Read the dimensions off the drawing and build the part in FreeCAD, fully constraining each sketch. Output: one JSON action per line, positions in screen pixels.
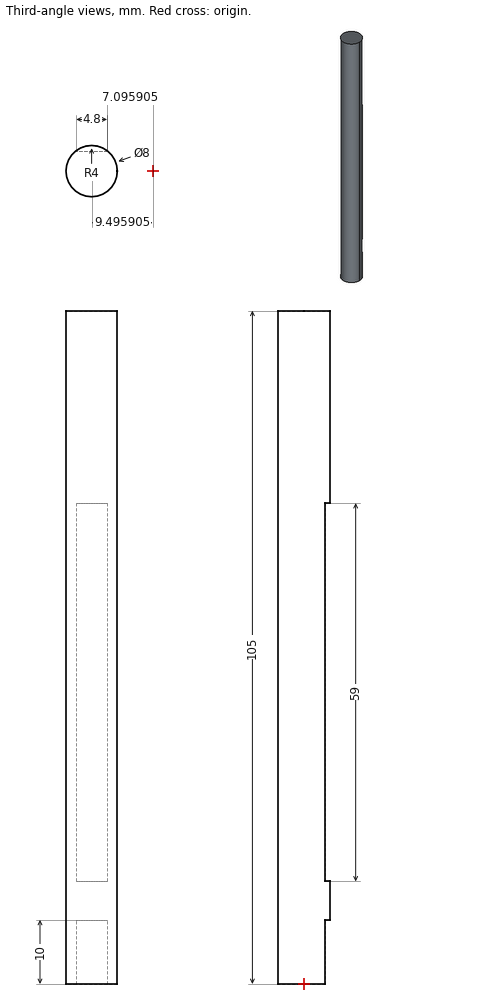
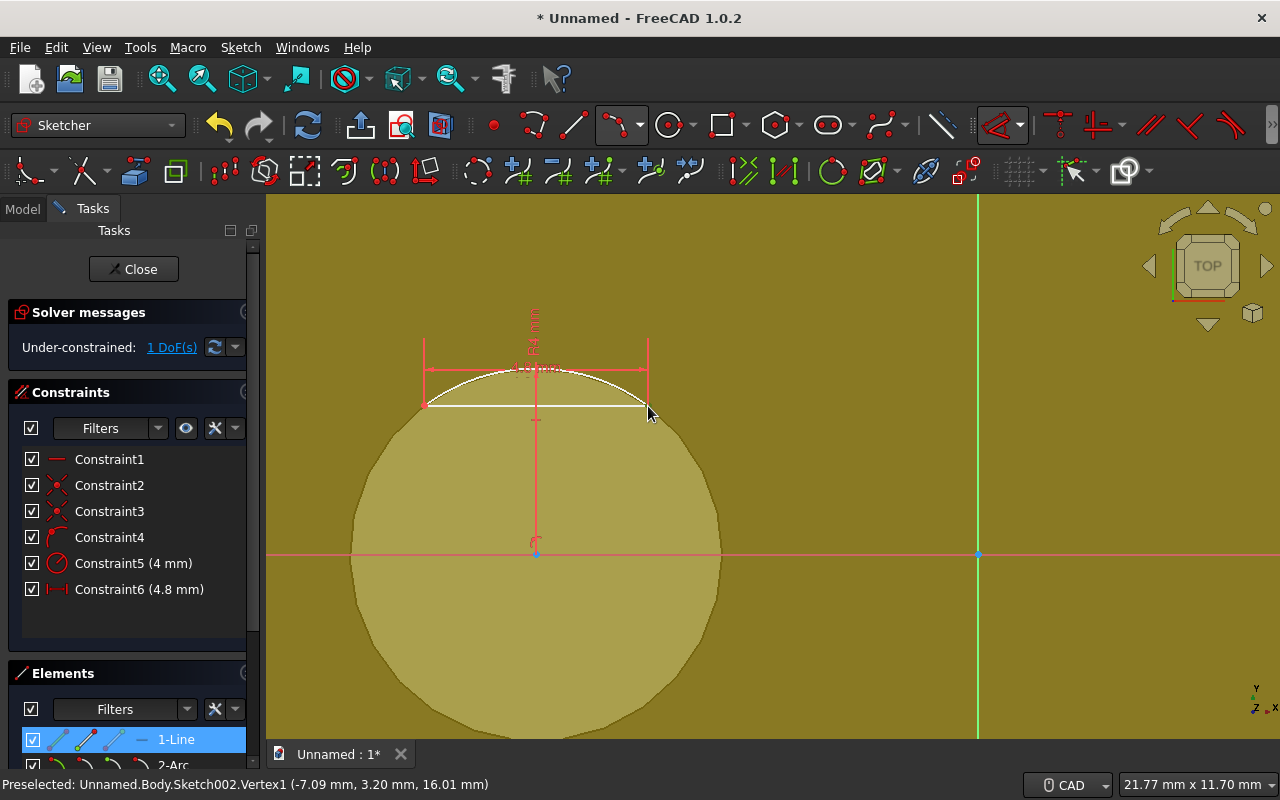
{"action": "key", "text": "l"}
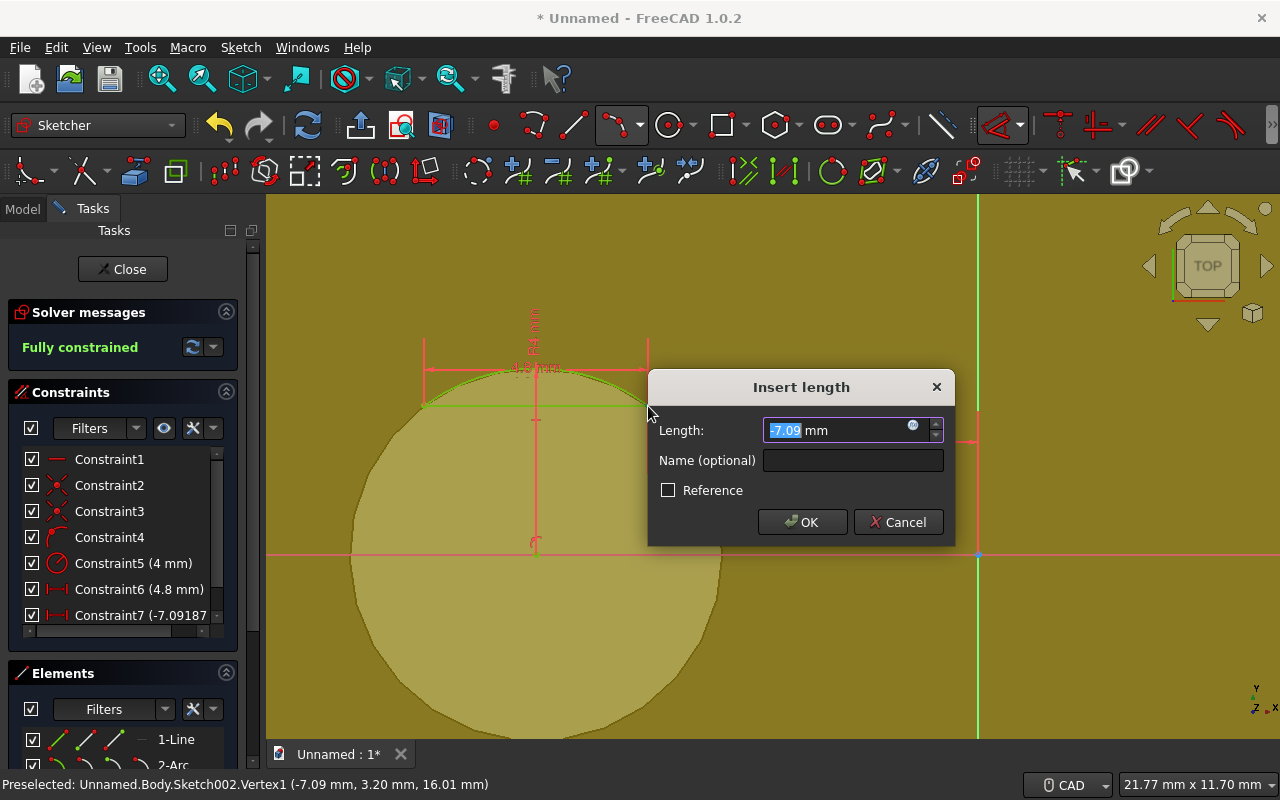
{"action": "type", "text": "-7.095905"}
{"action": "key", "text": "Return"}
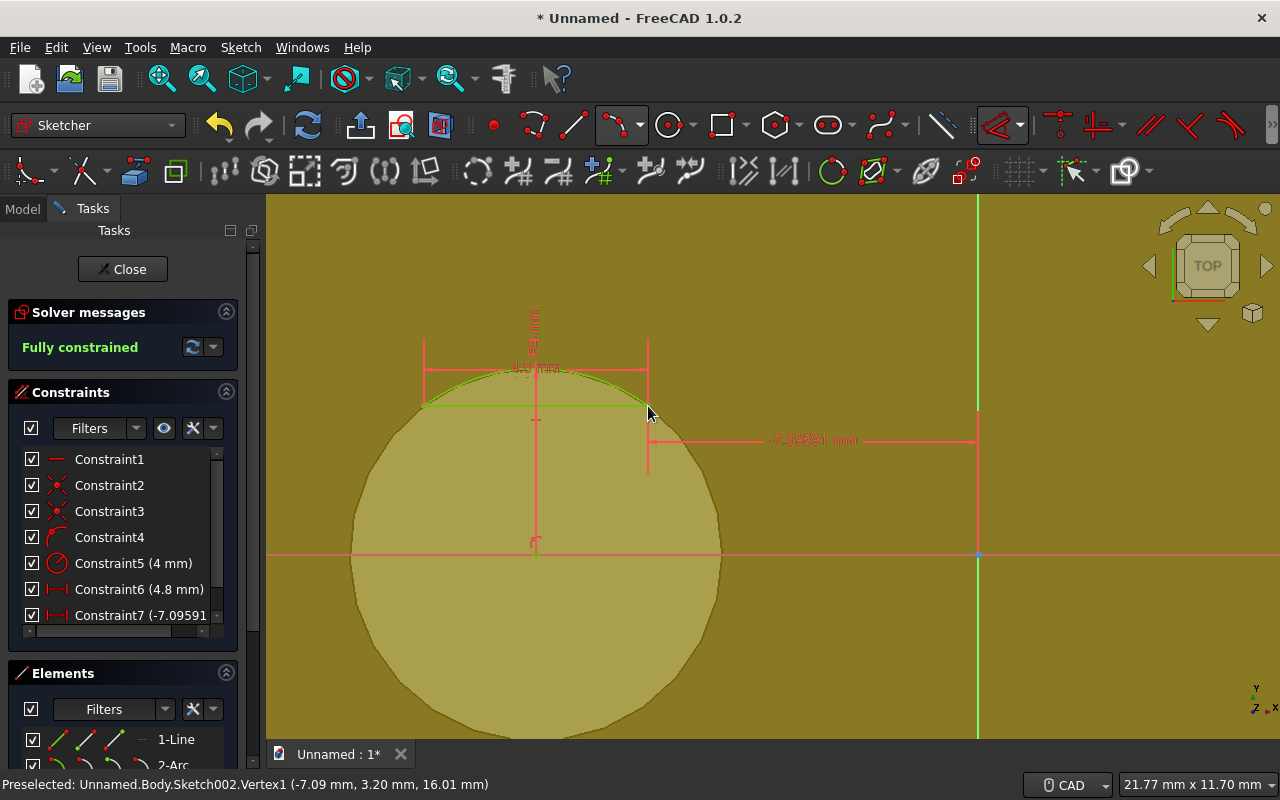
{"action": "left_click", "coordinate": [123, 269]}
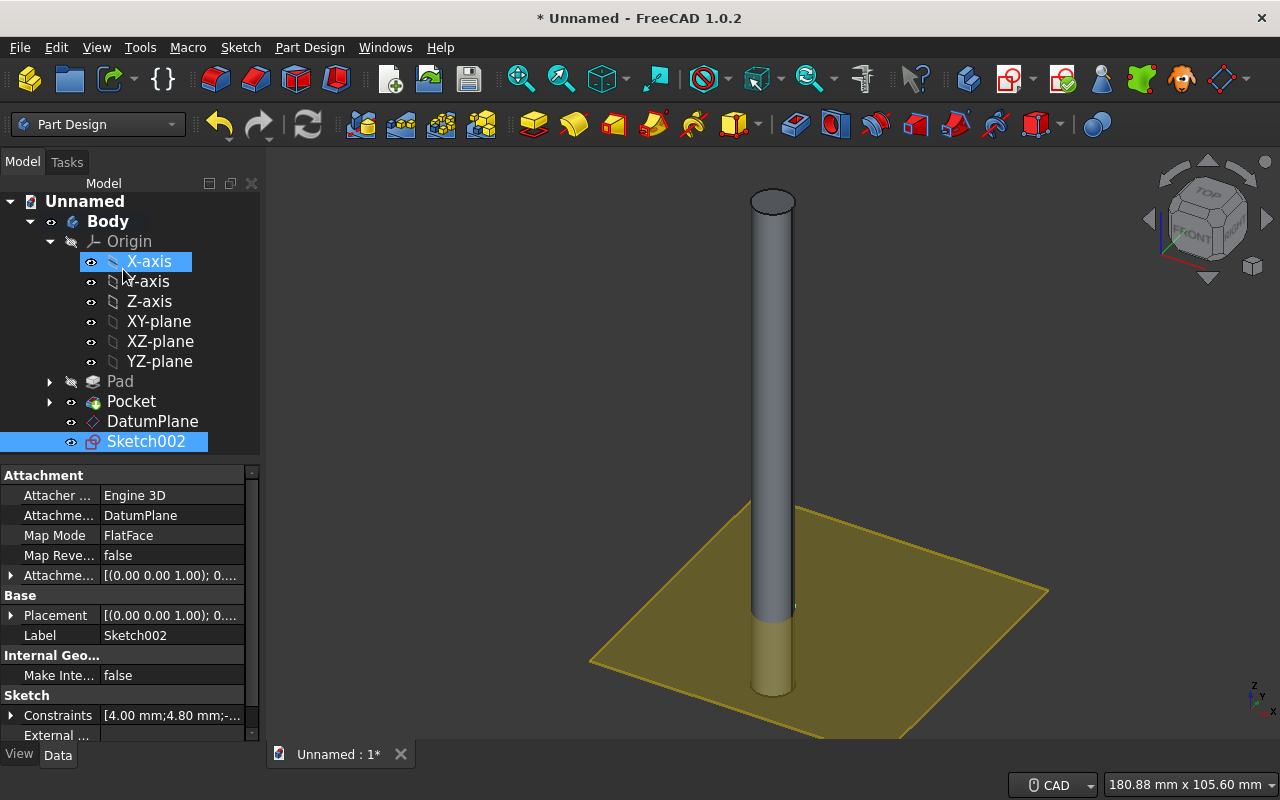
{"action": "left_click", "coordinate": [796, 124]}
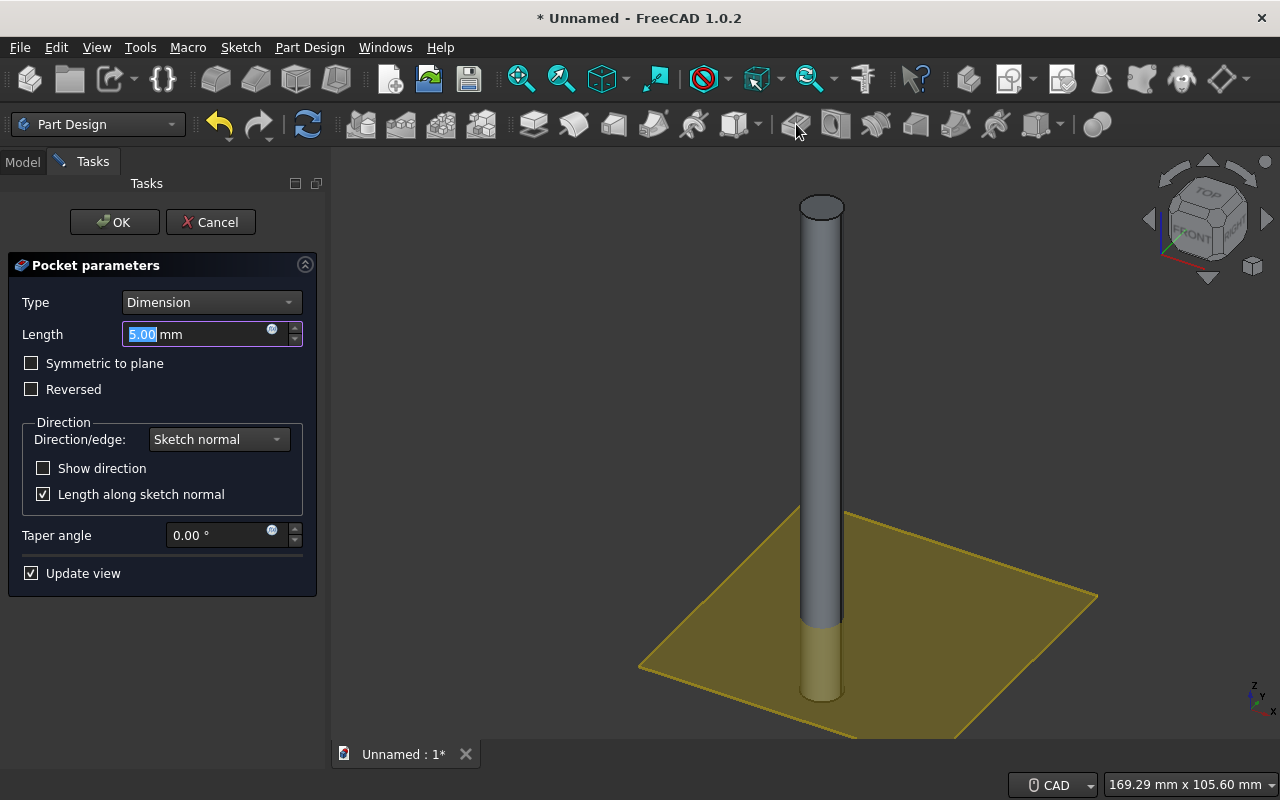
{"action": "type", "text": "59"}
{"action": "key", "text": "Tab"}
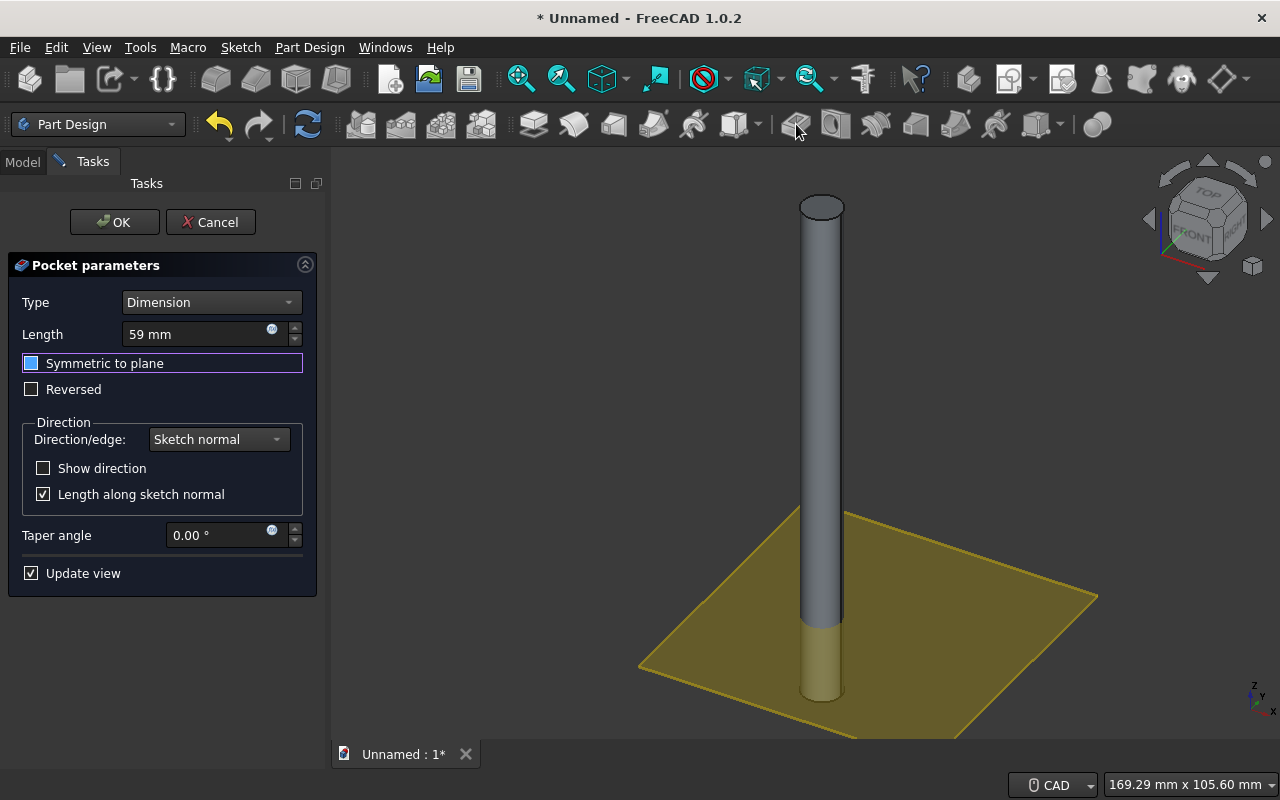
{"action": "left_click", "coordinate": [30, 389]}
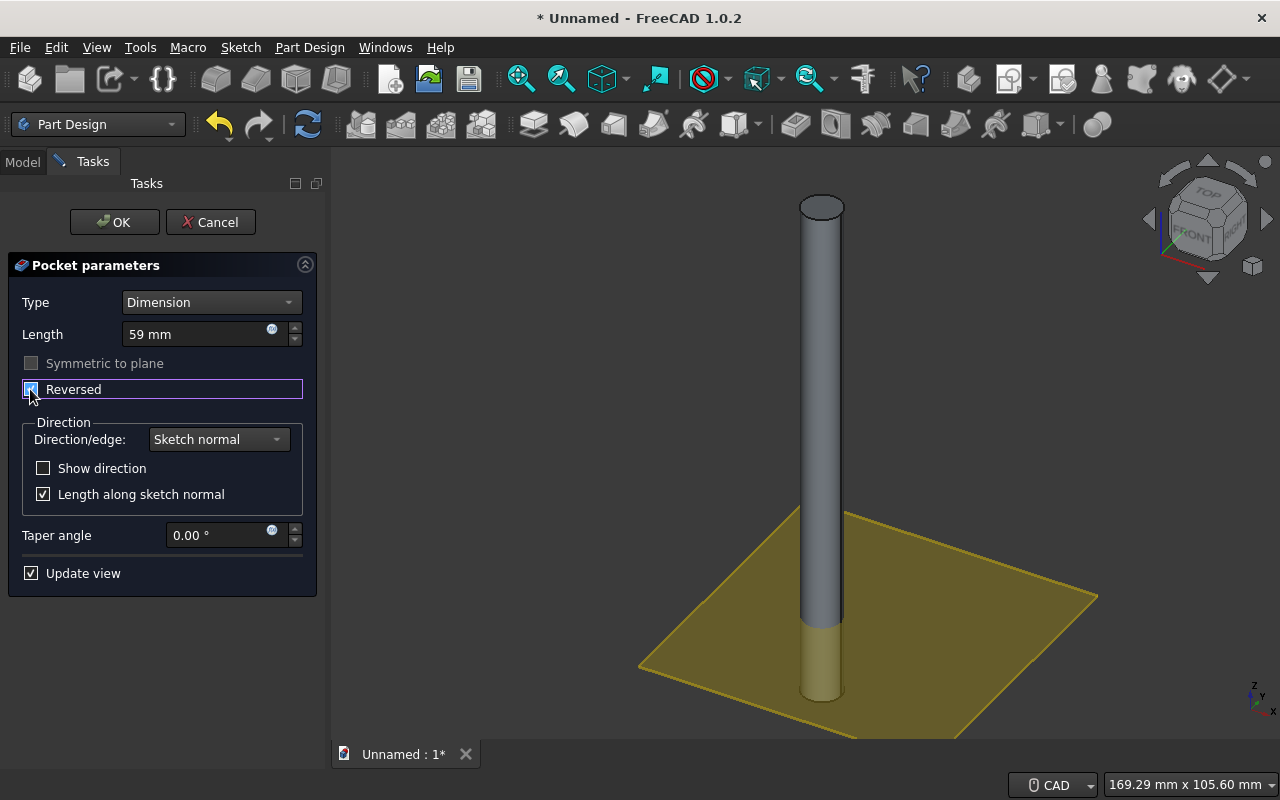
{"action": "left_click", "coordinate": [115, 222]}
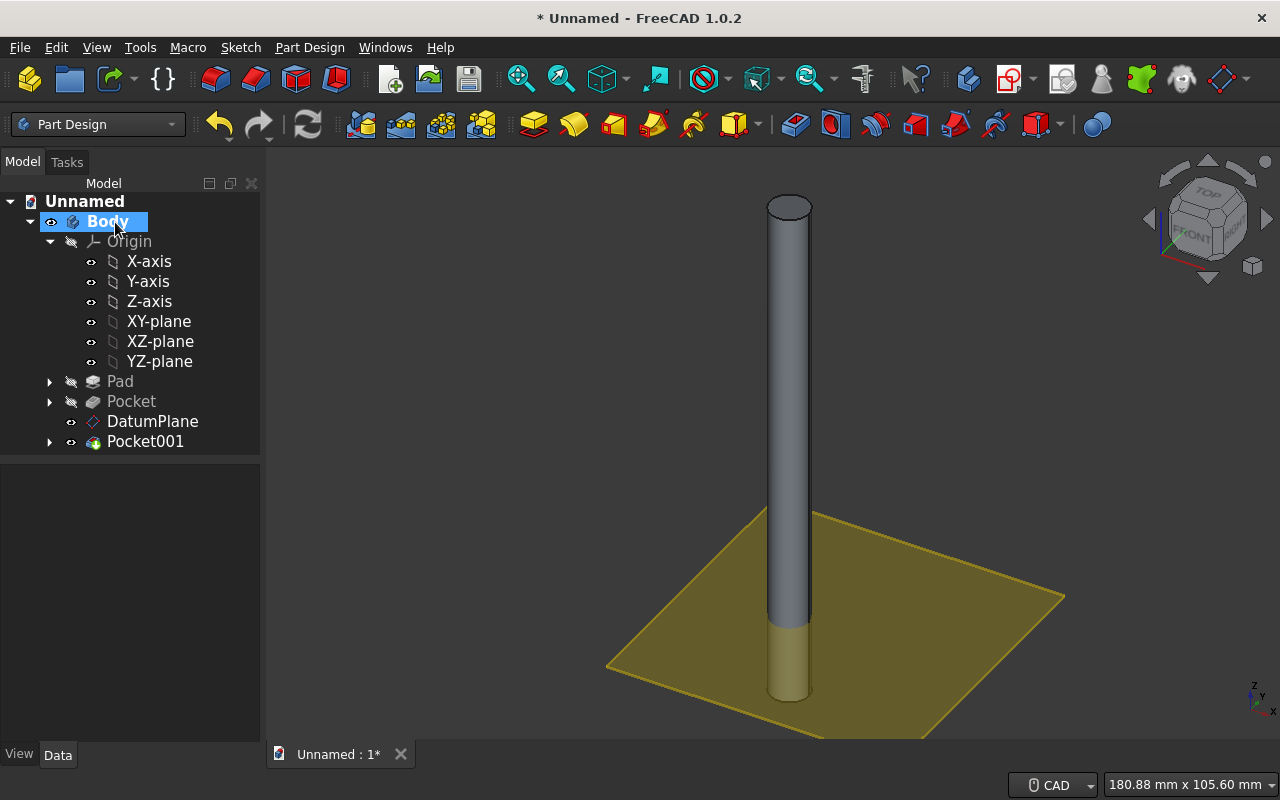
{"action": "left_click", "coordinate": [116, 422]}
{"action": "key", "text": "space"}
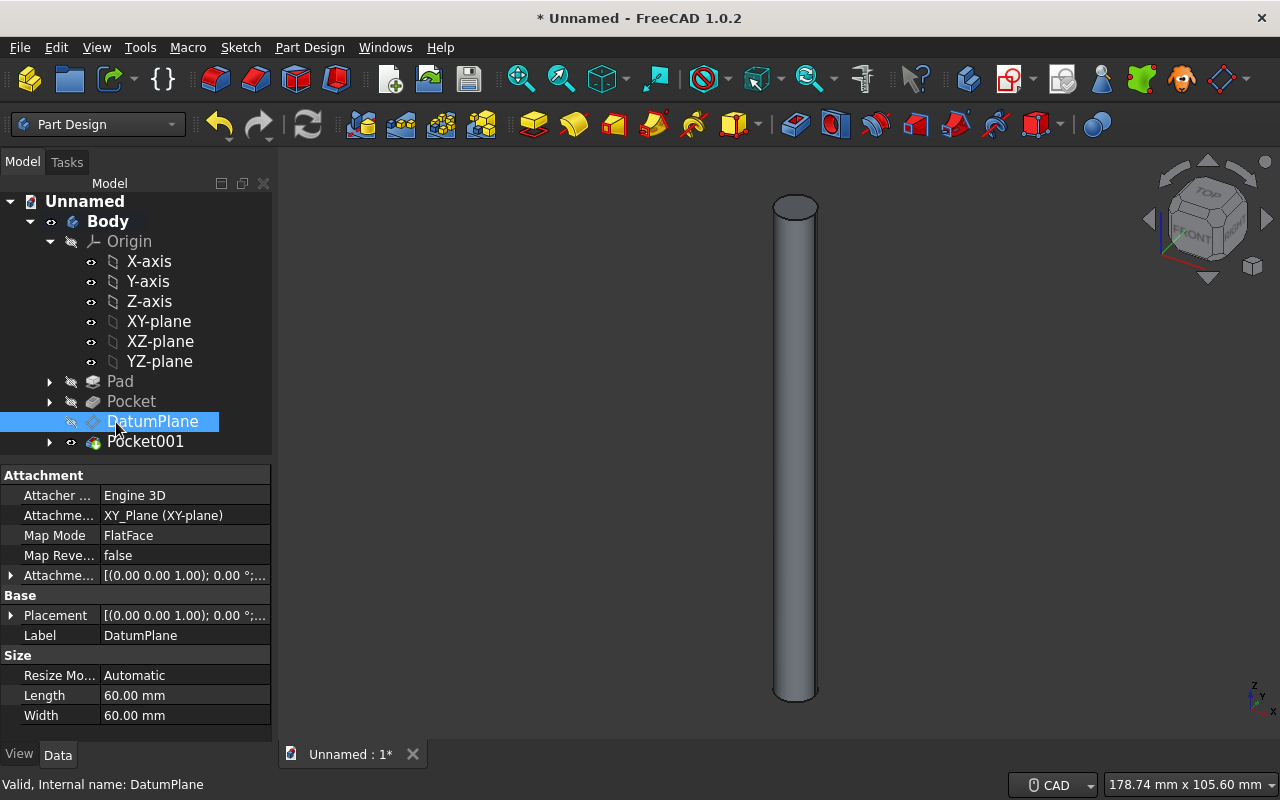
{"action": "key", "text": "0"}